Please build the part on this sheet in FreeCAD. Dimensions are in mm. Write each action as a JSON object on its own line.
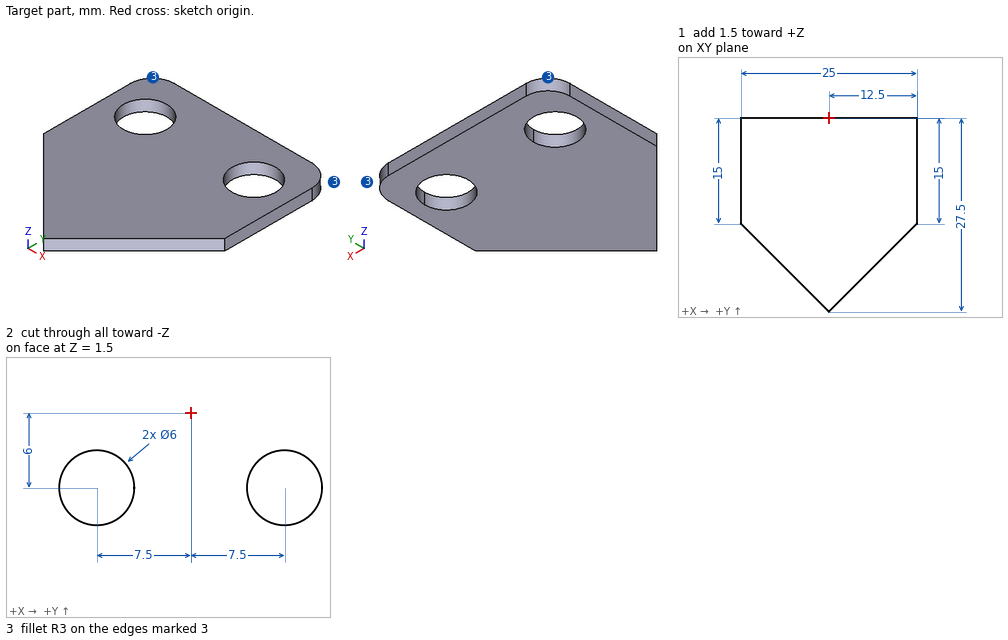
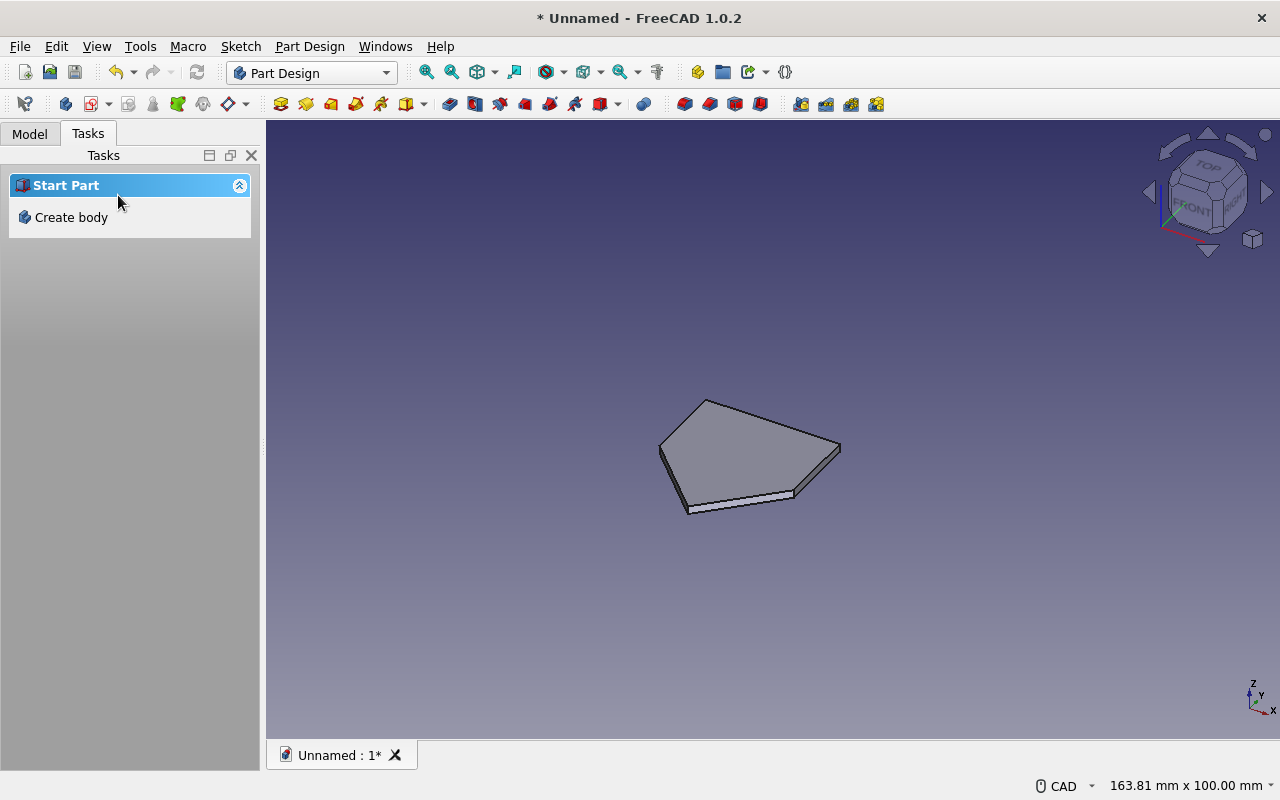
{"action": "left_click", "coordinate": [427, 72]}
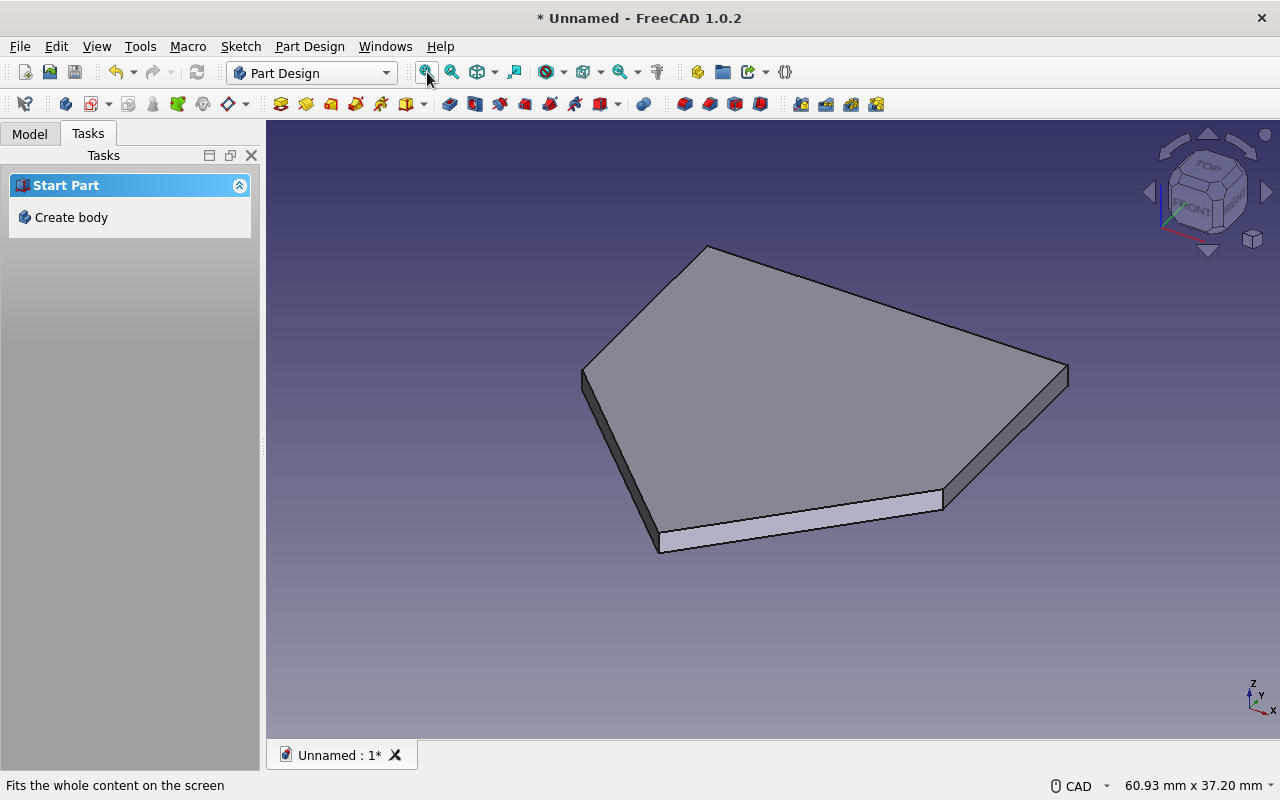
{"action": "left_click", "coordinate": [806, 386]}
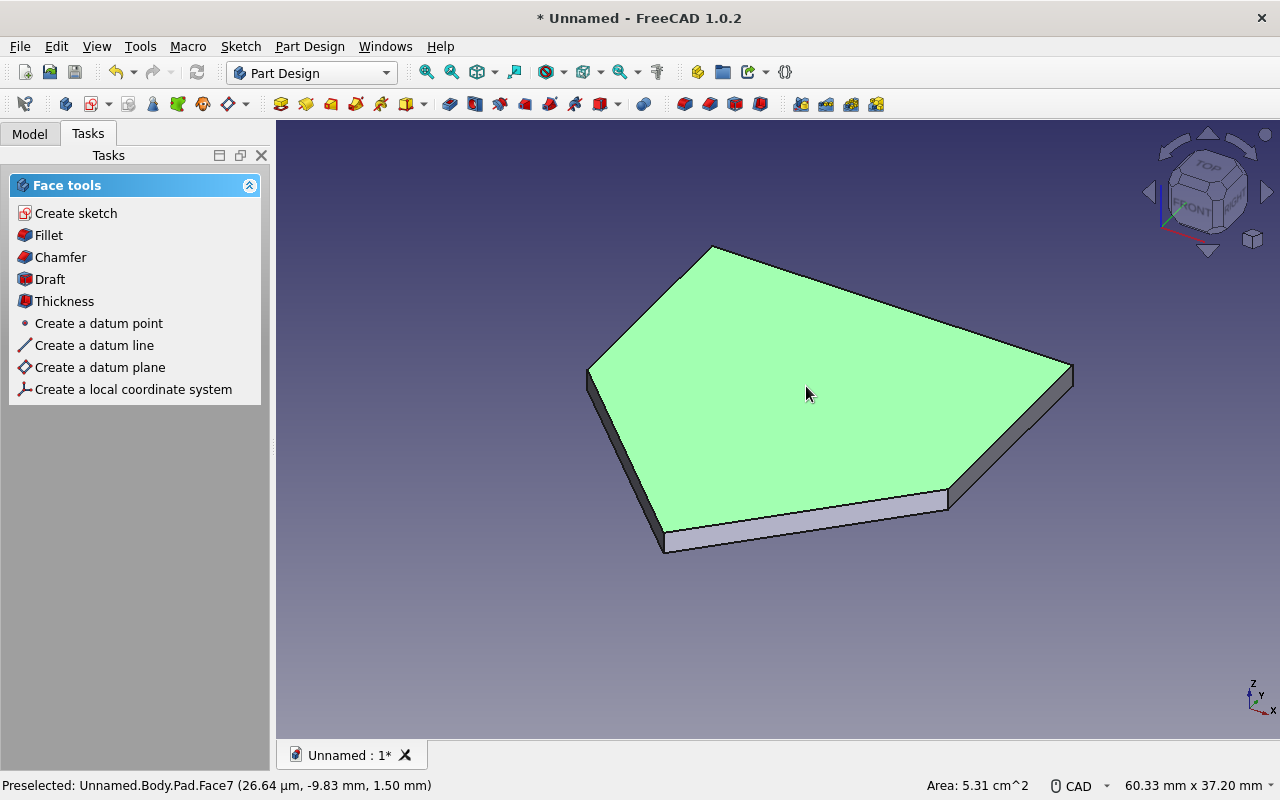
{"action": "left_click", "coordinate": [90, 104]}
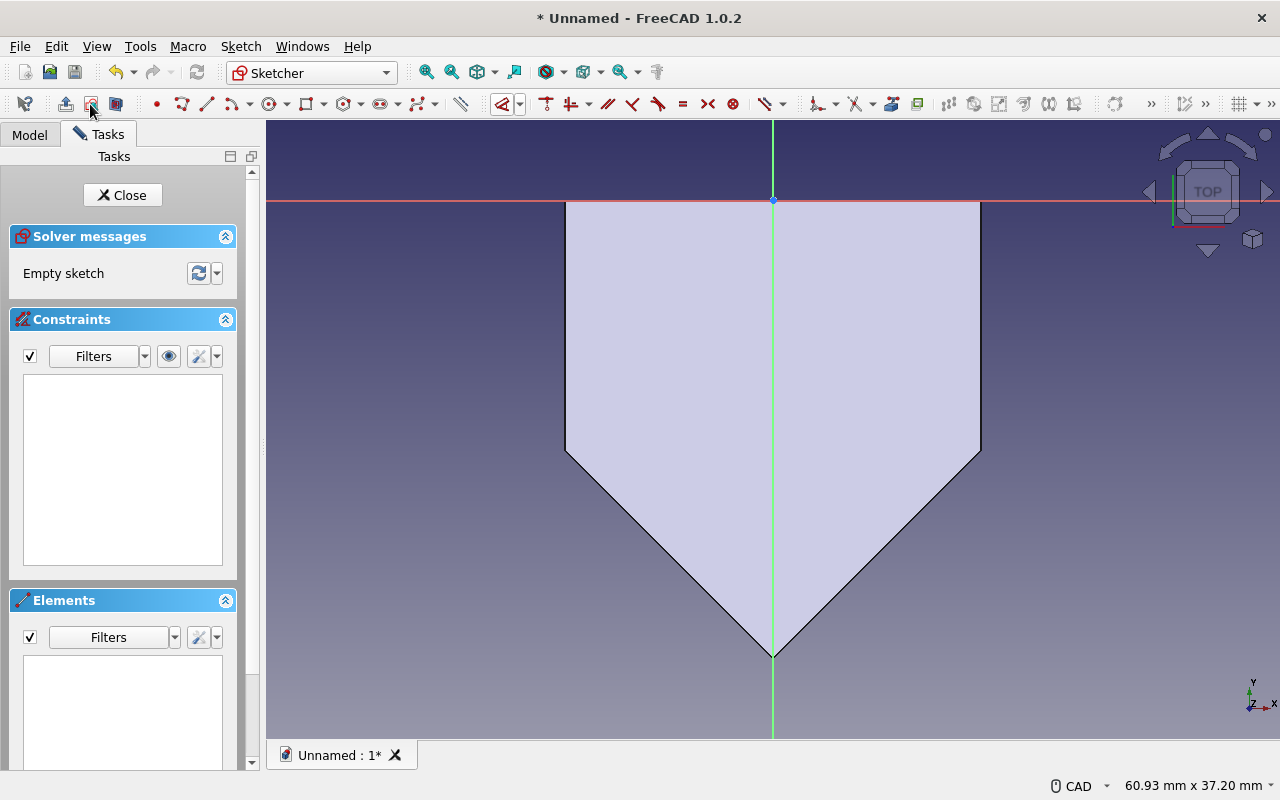
{"action": "scroll", "coordinate": [856, 148], "scroll_direction": "up", "scroll_amount": 3}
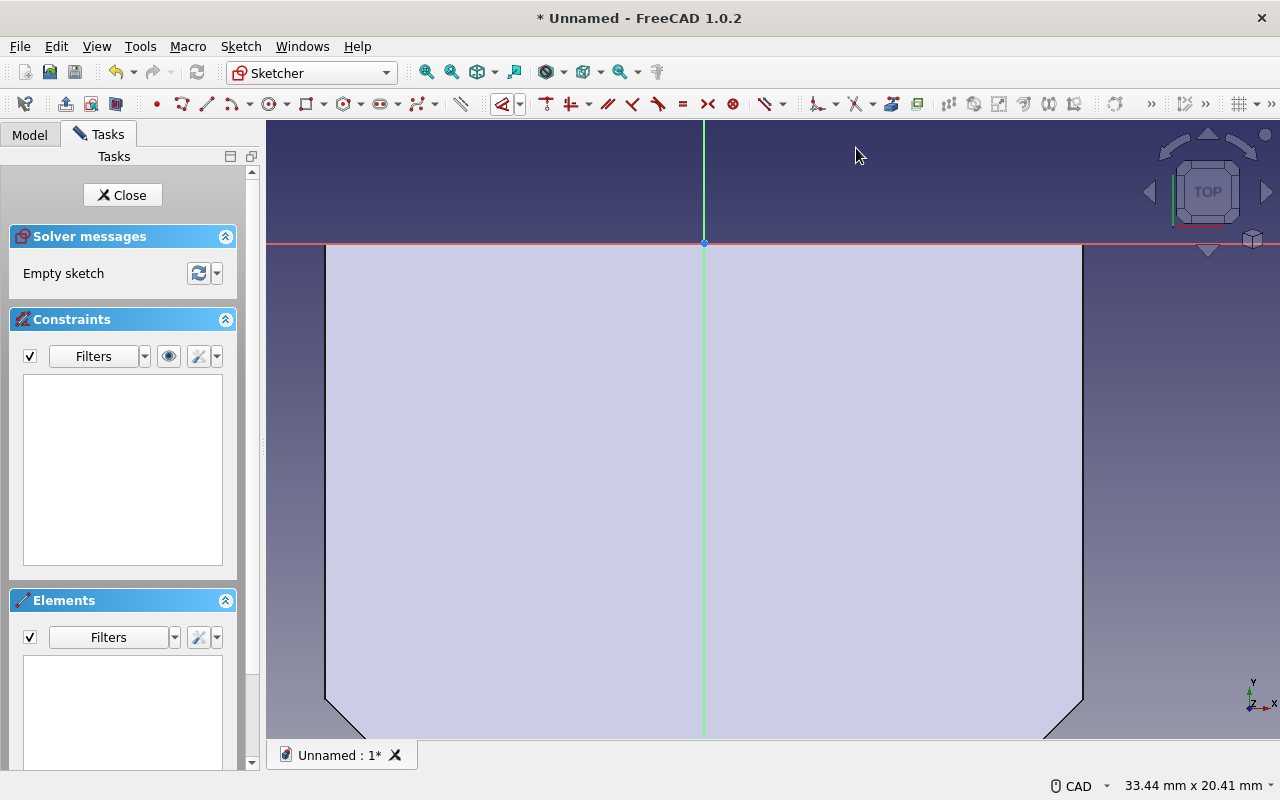
{"action": "left_click", "coordinate": [268, 104]}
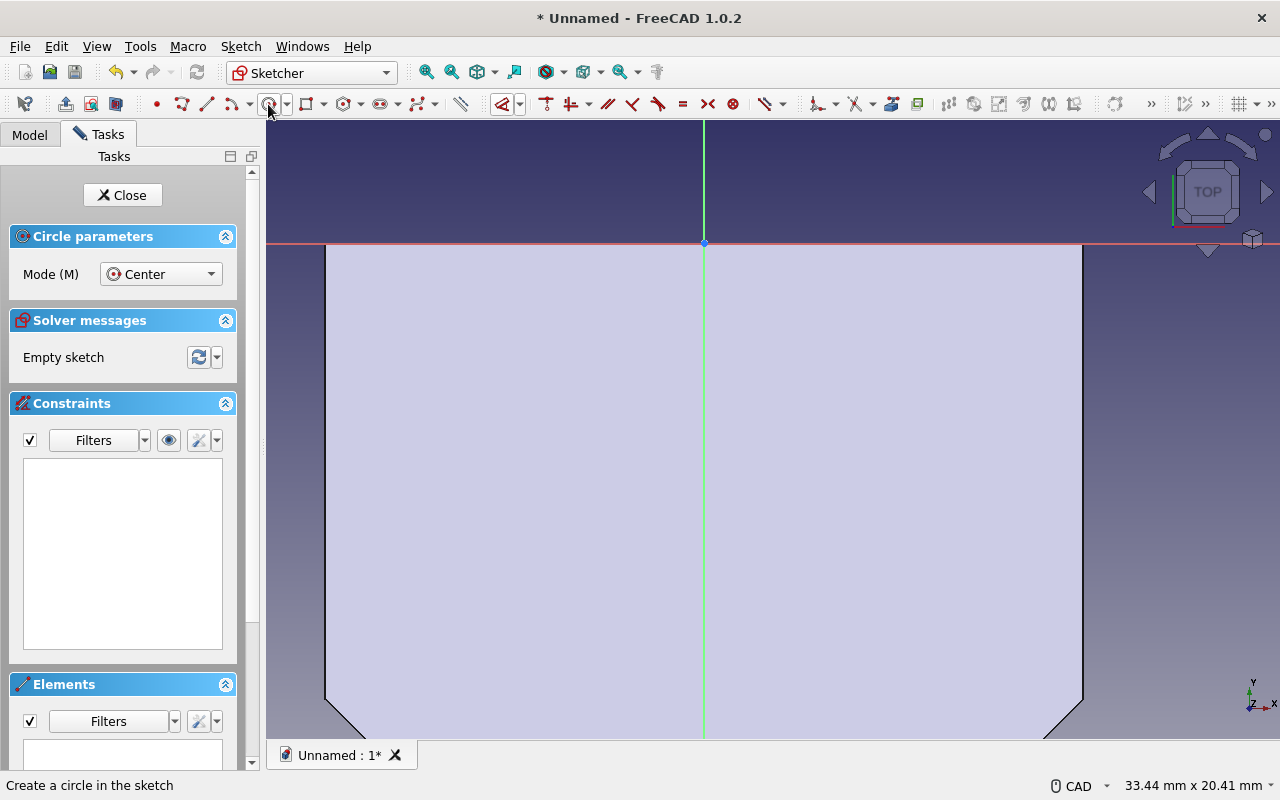
{"action": "left_click", "coordinate": [477, 426]}
{"action": "left_click", "coordinate": [541, 362]}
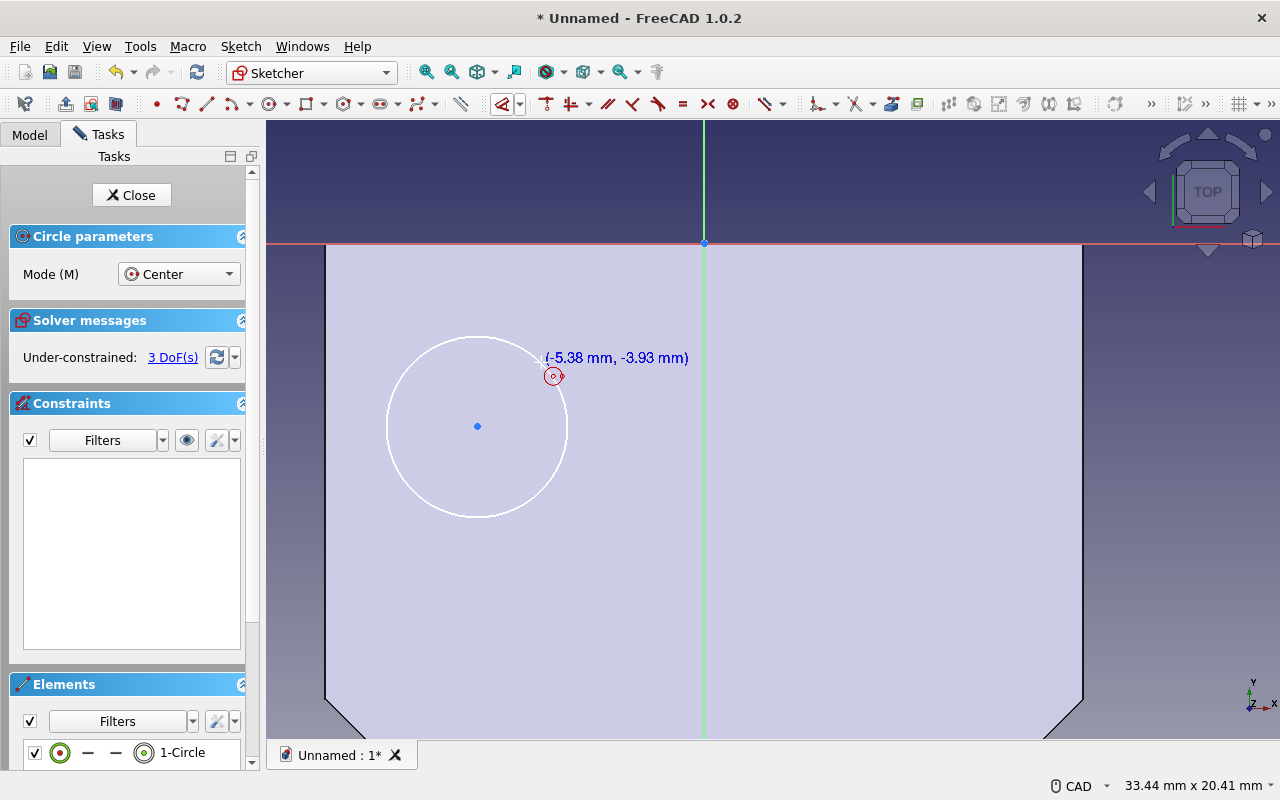
{"action": "left_click", "coordinate": [932, 426]}
{"action": "left_click", "coordinate": [996, 362]}
{"action": "key", "text": "Escape"}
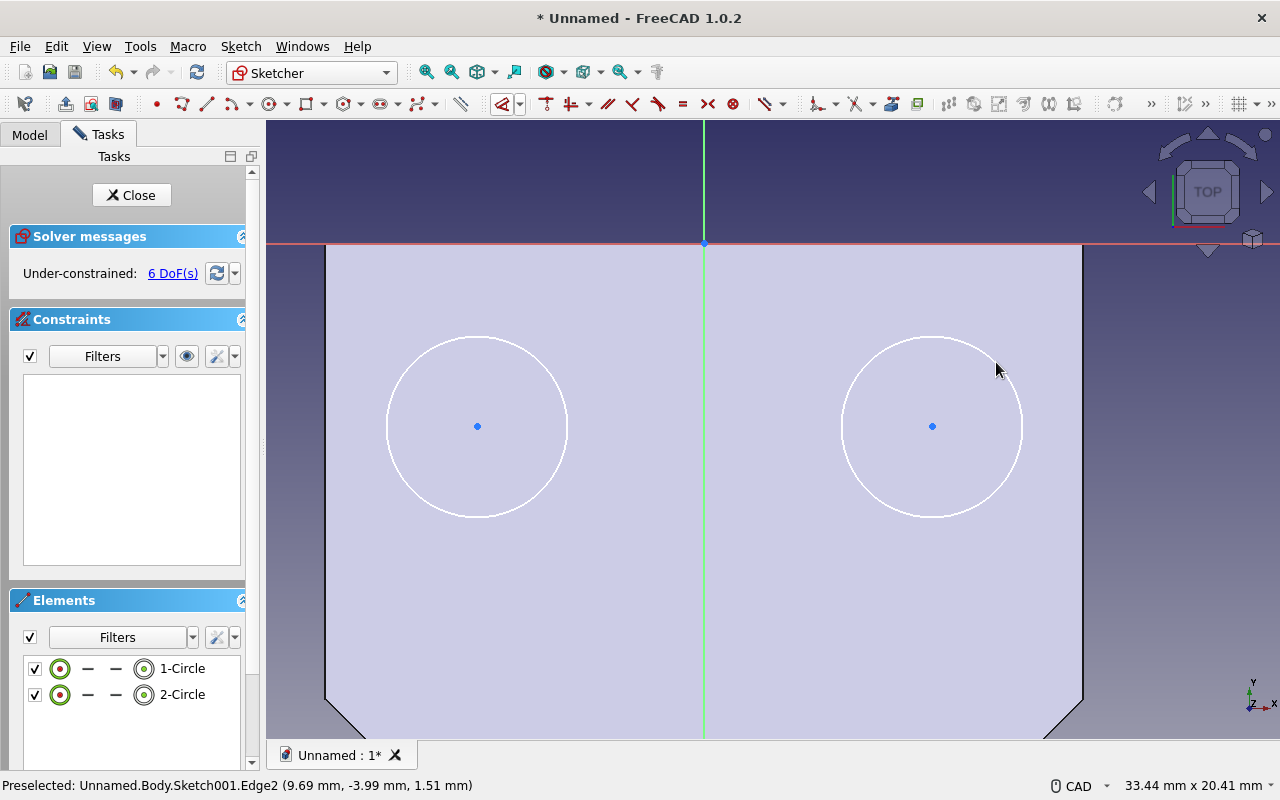
{"action": "left_click", "coordinate": [541, 363]}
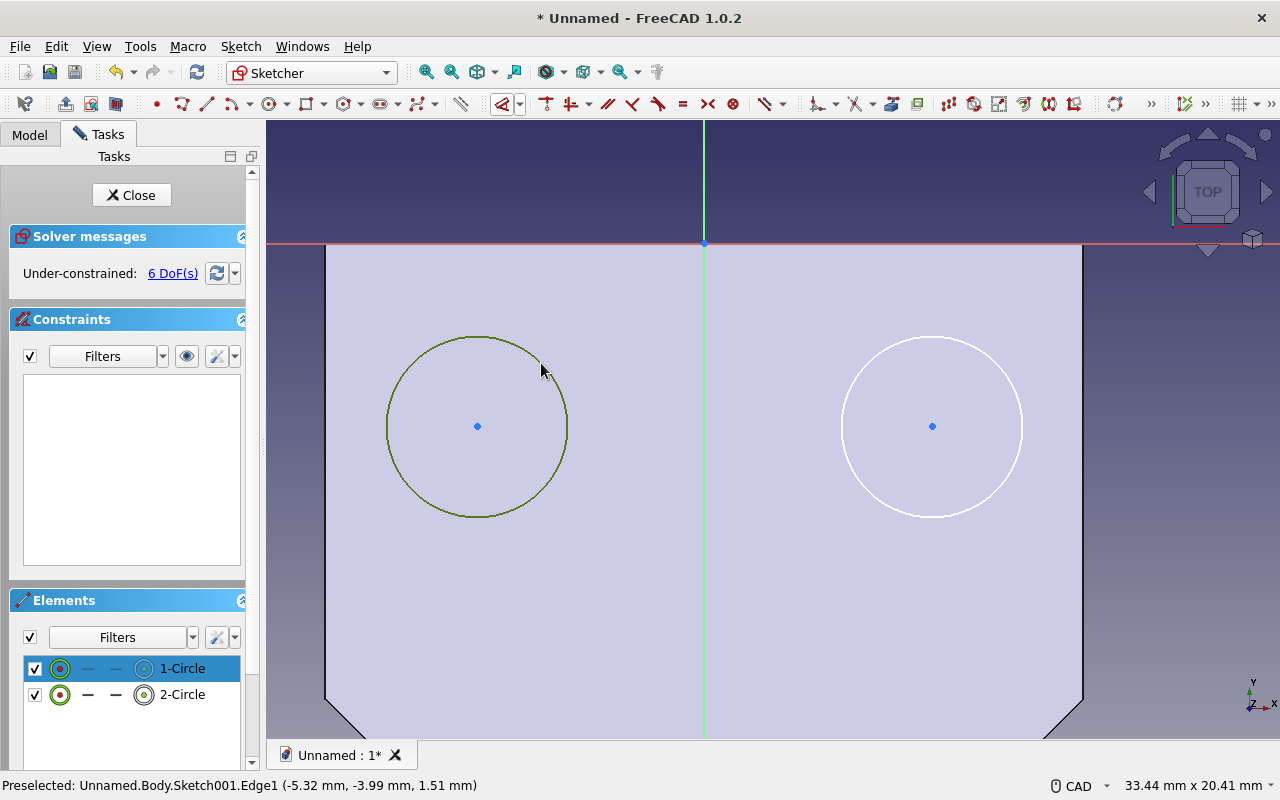
{"action": "left_click", "coordinate": [996, 363]}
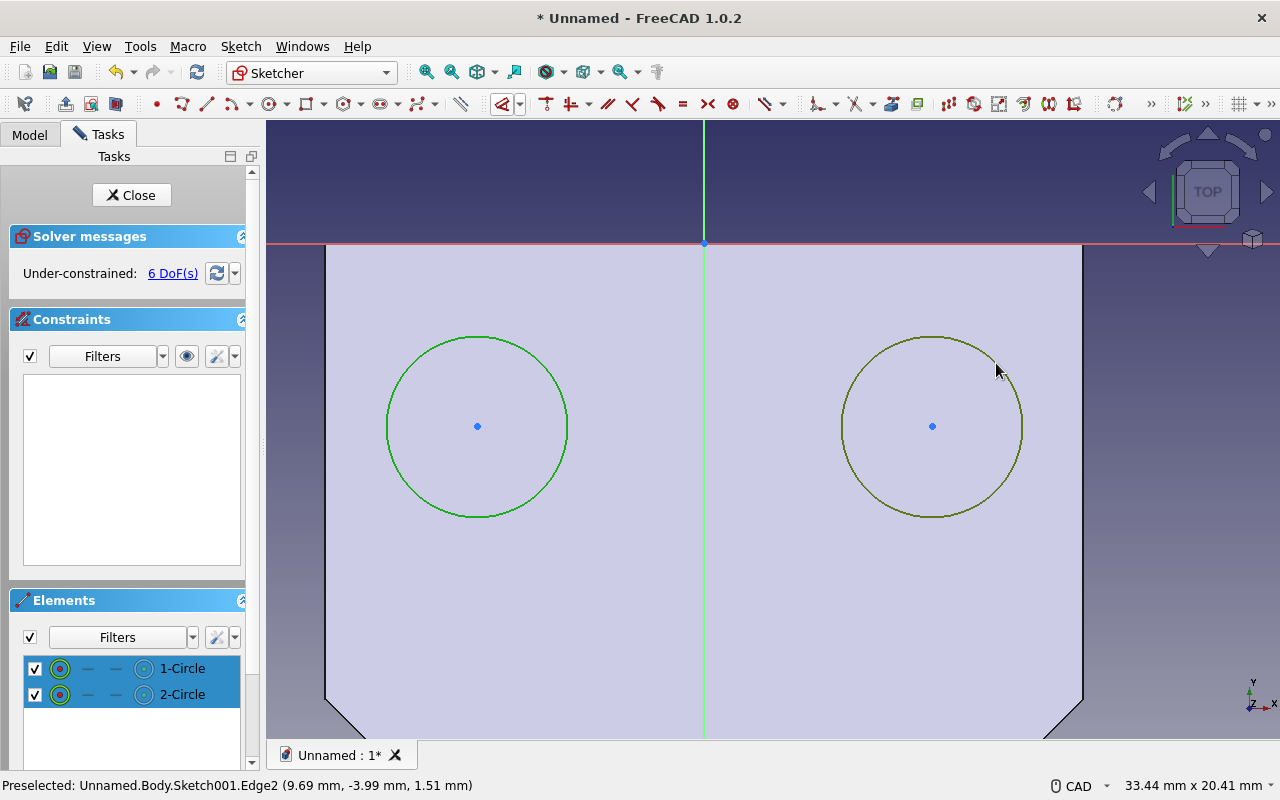
{"action": "left_click", "coordinate": [683, 104]}